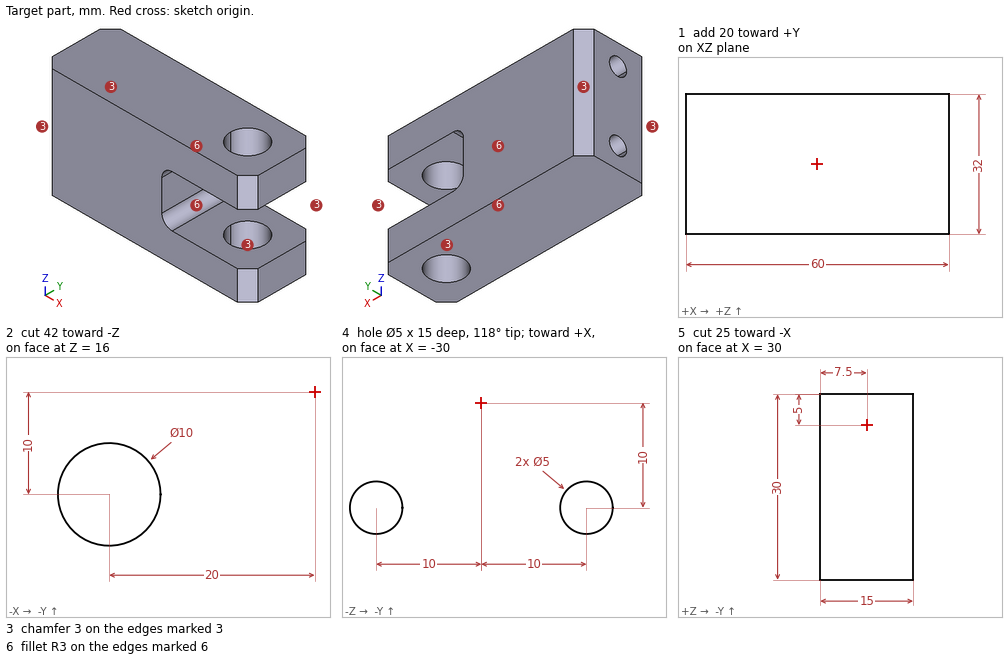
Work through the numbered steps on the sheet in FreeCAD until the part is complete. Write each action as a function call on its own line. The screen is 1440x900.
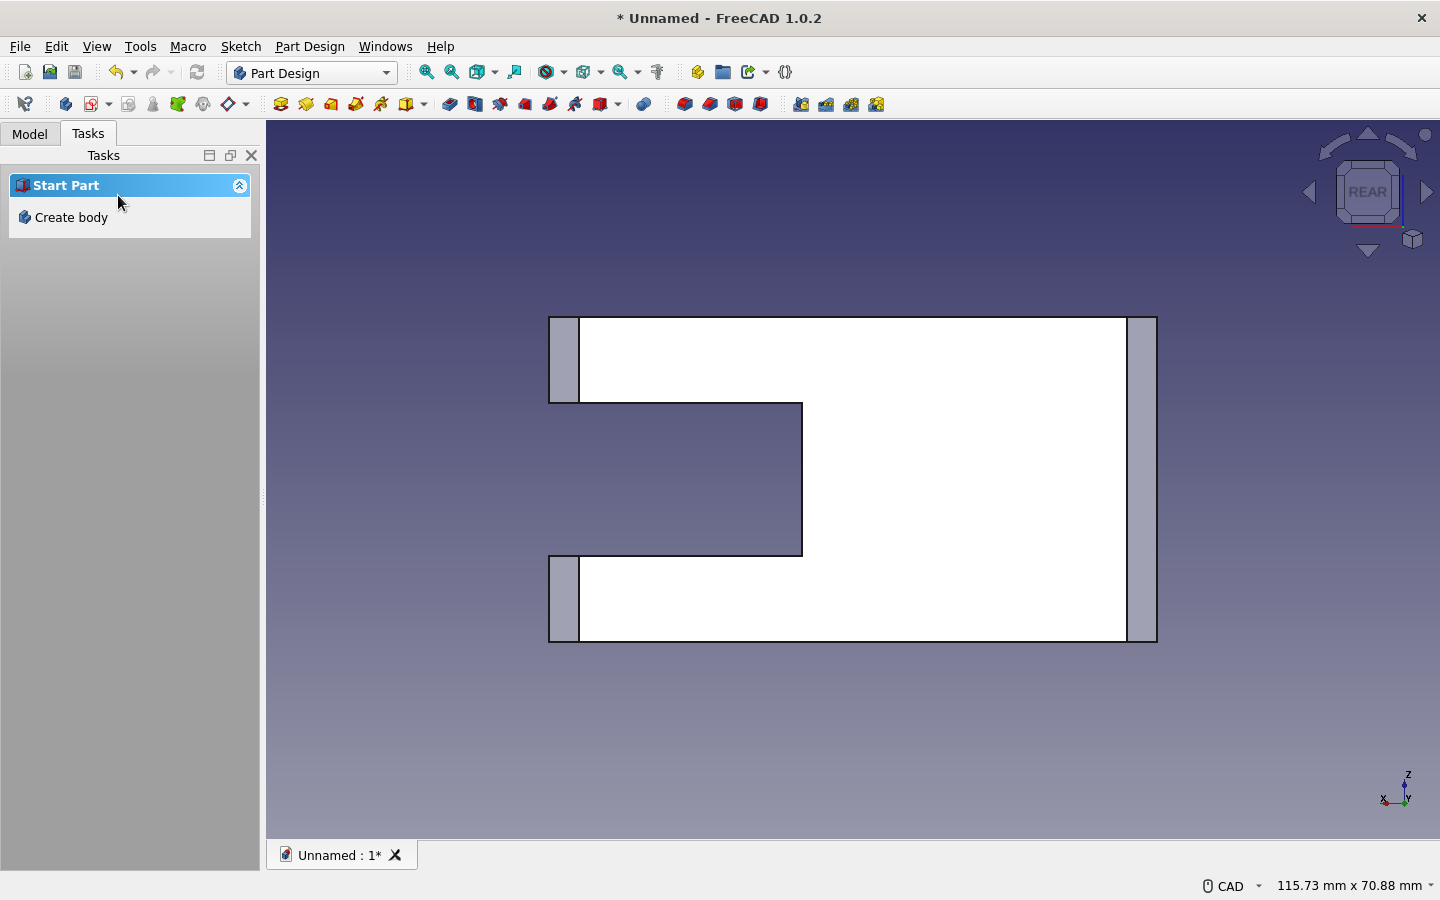
key(6)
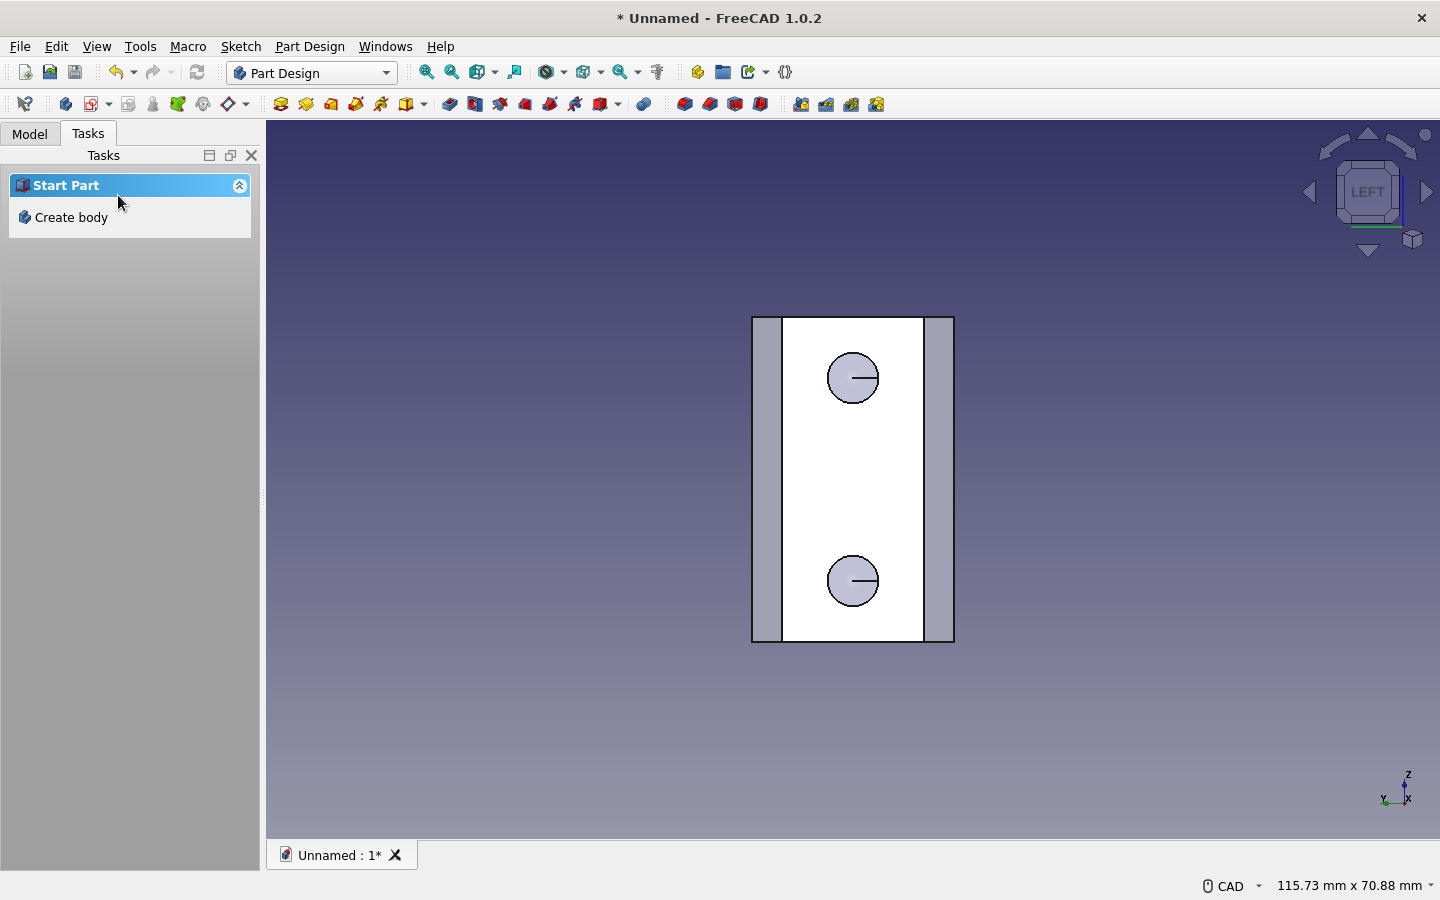
key(v)
key(3)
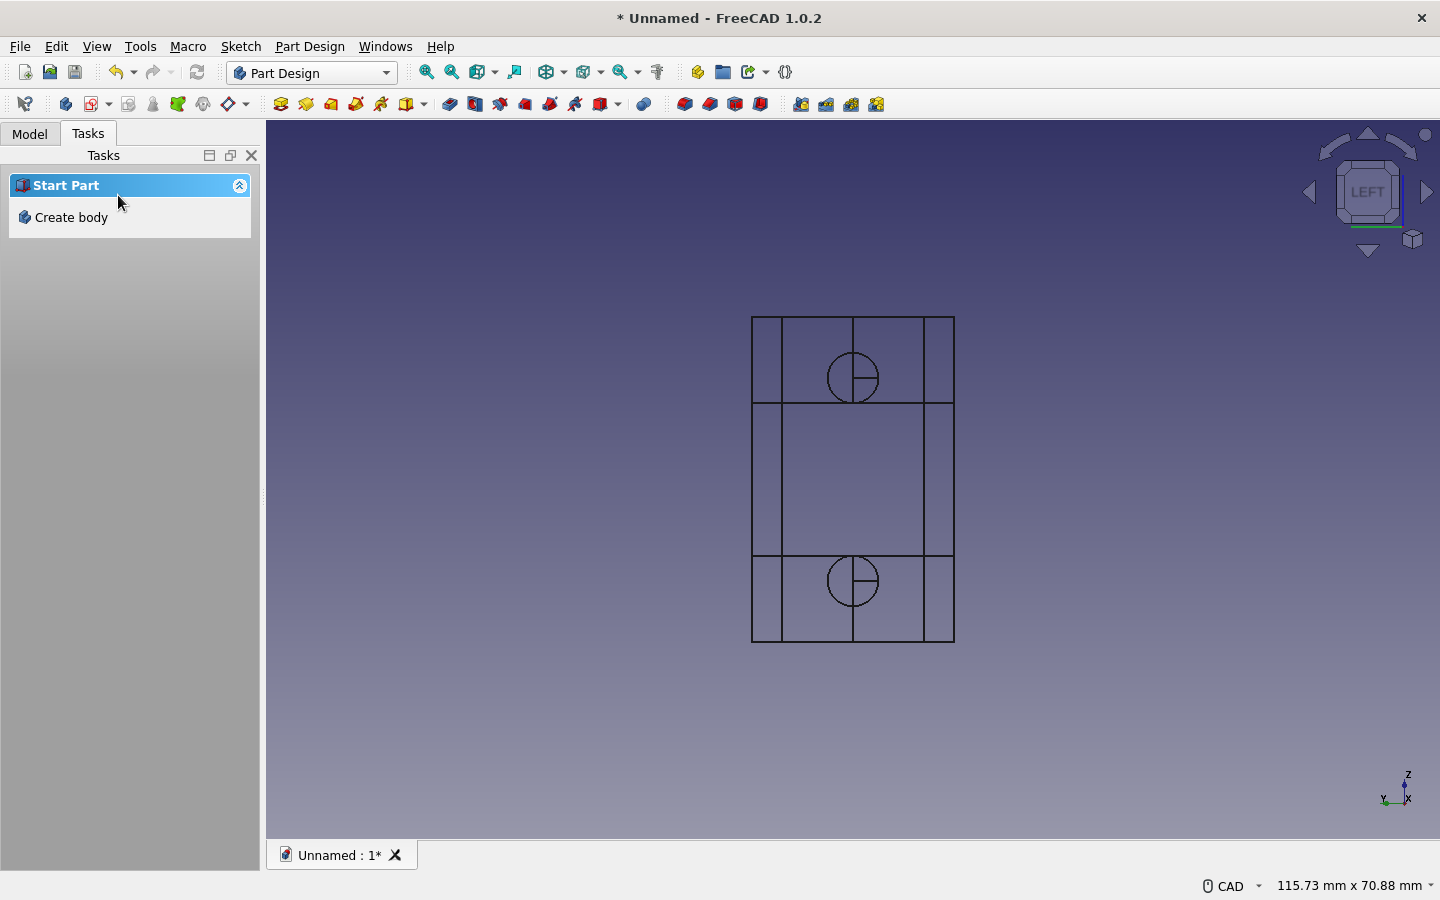
key(0)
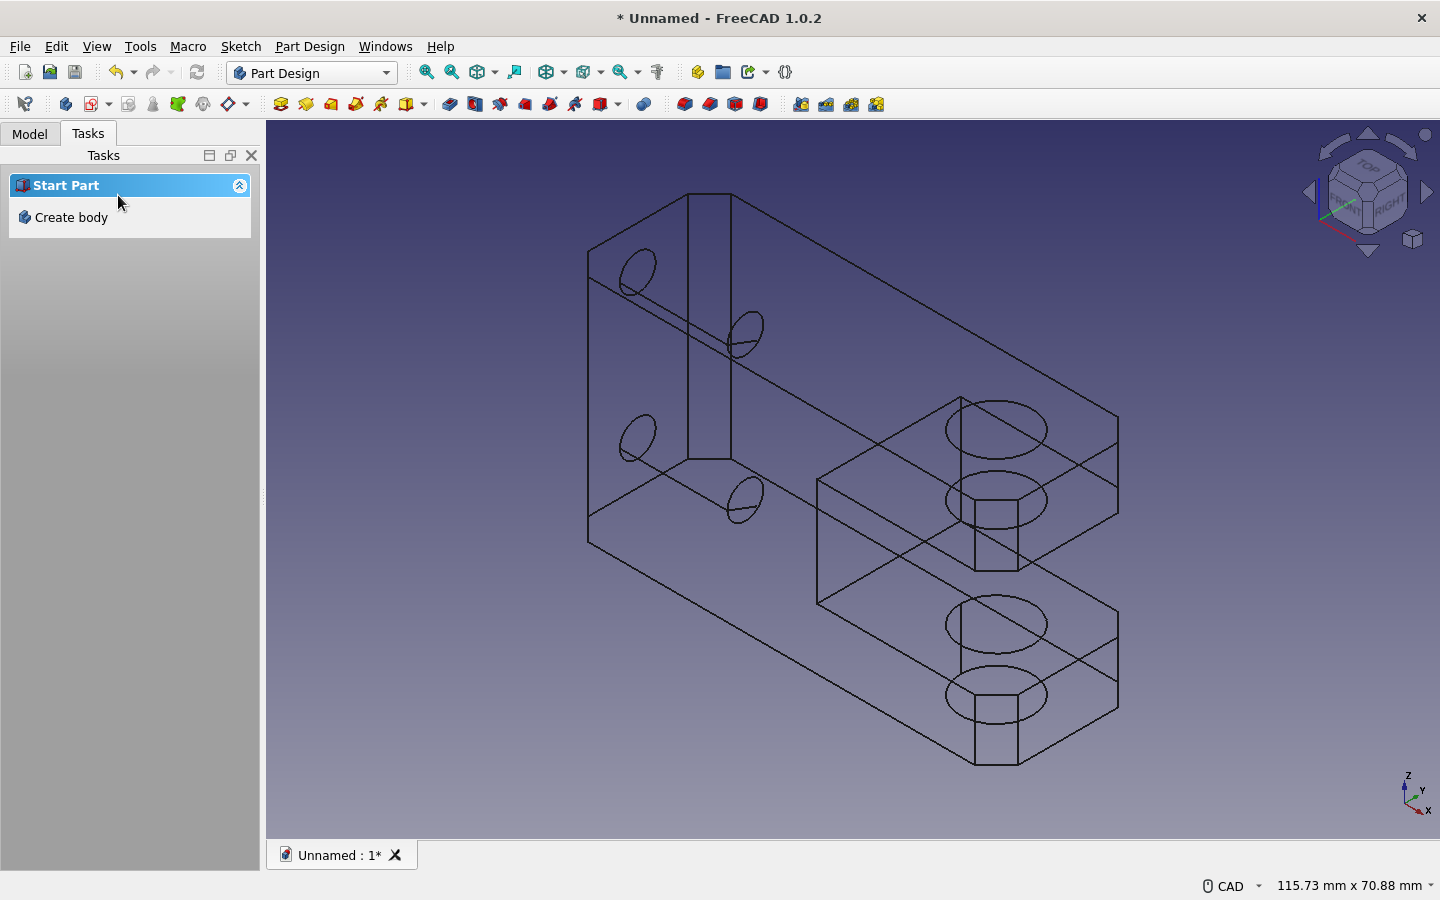
click(889, 561)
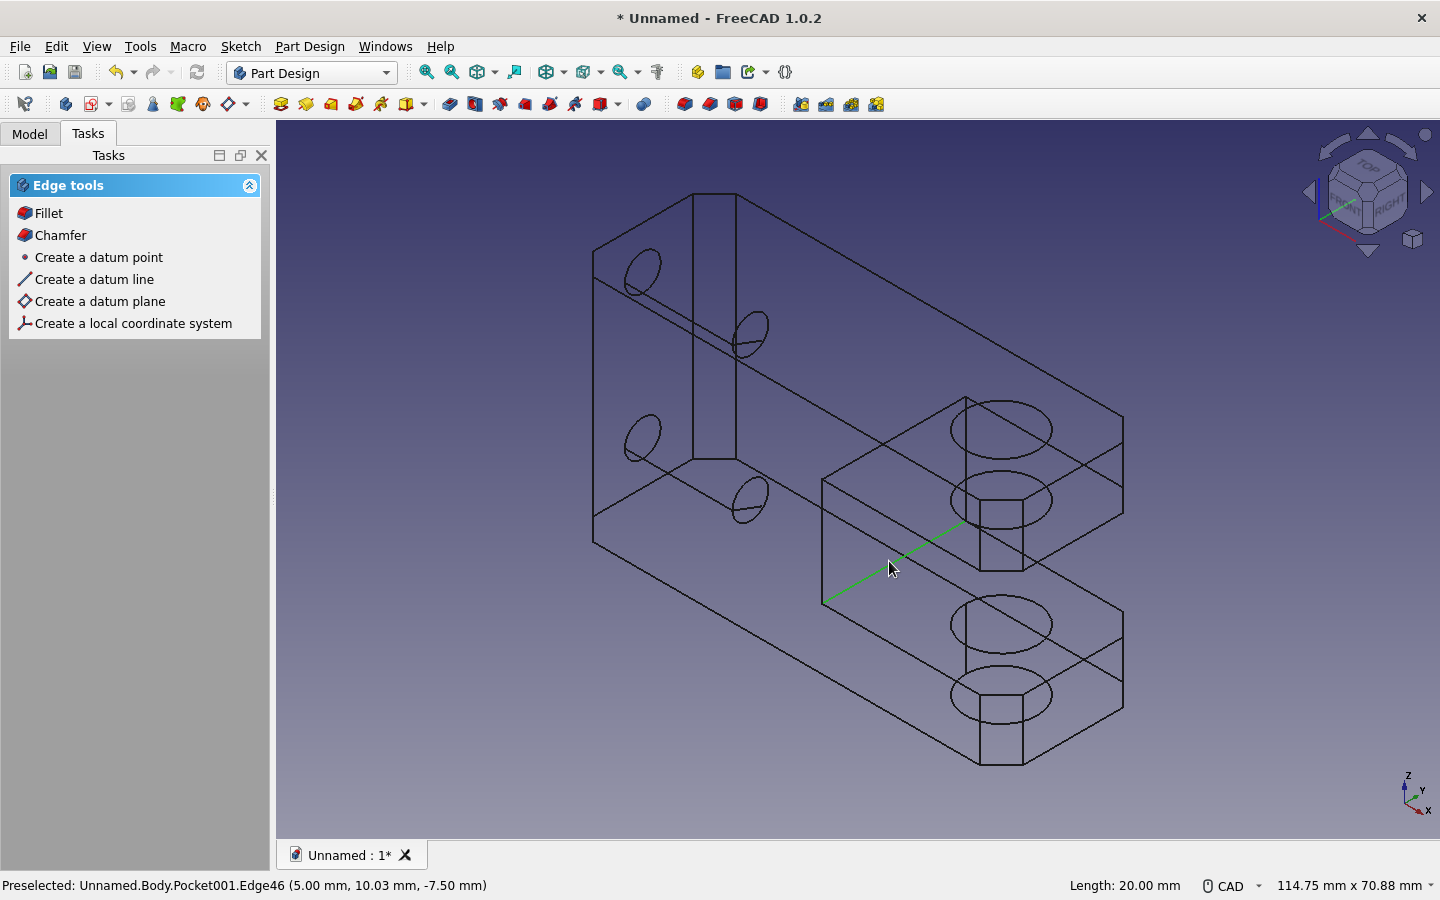
click(894, 437, ctrl)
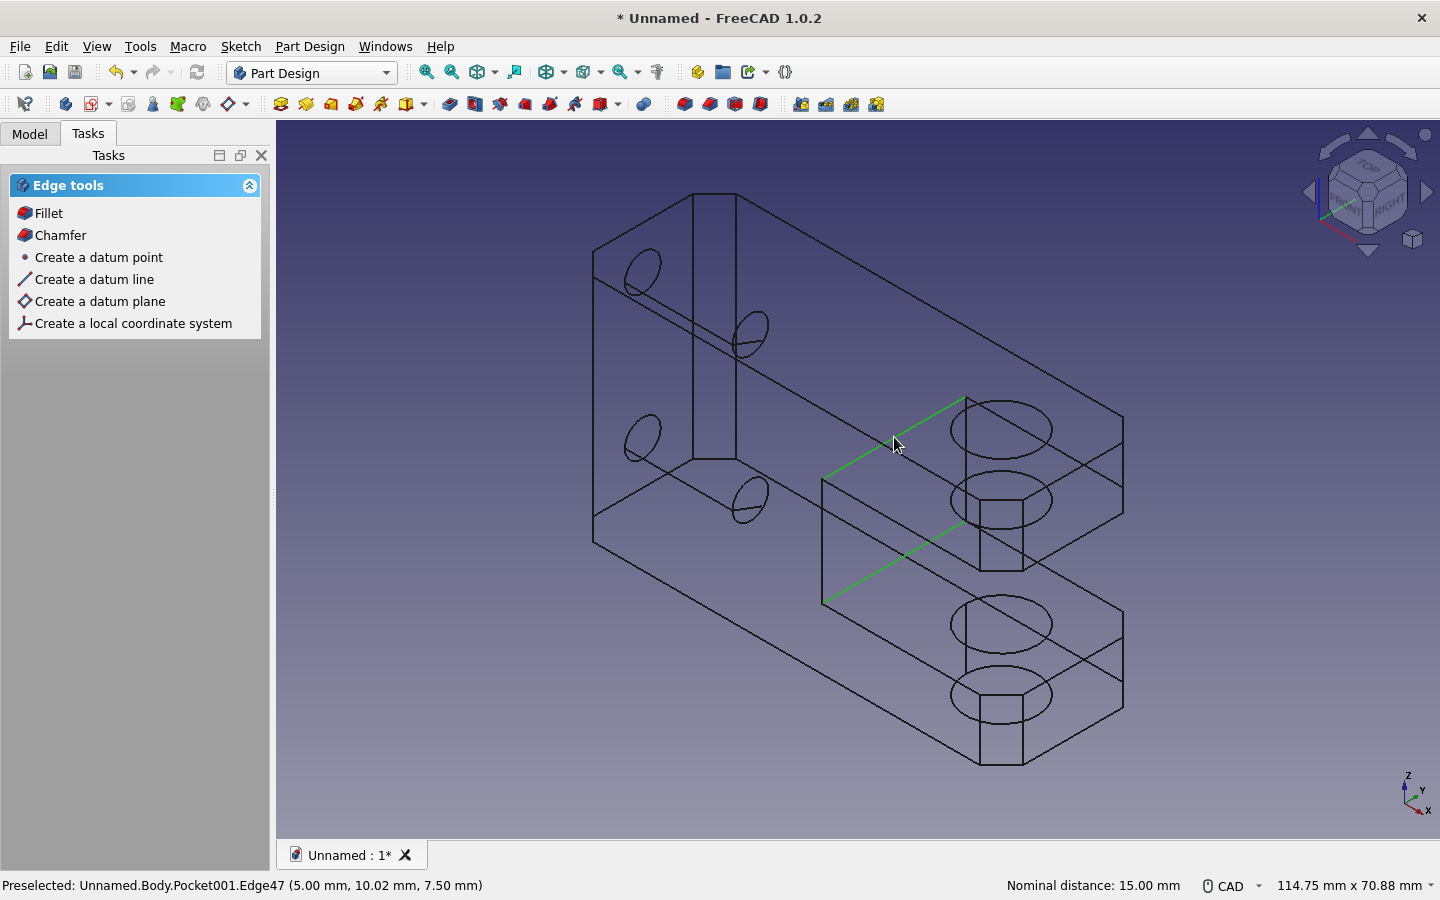
key(v)
key(1)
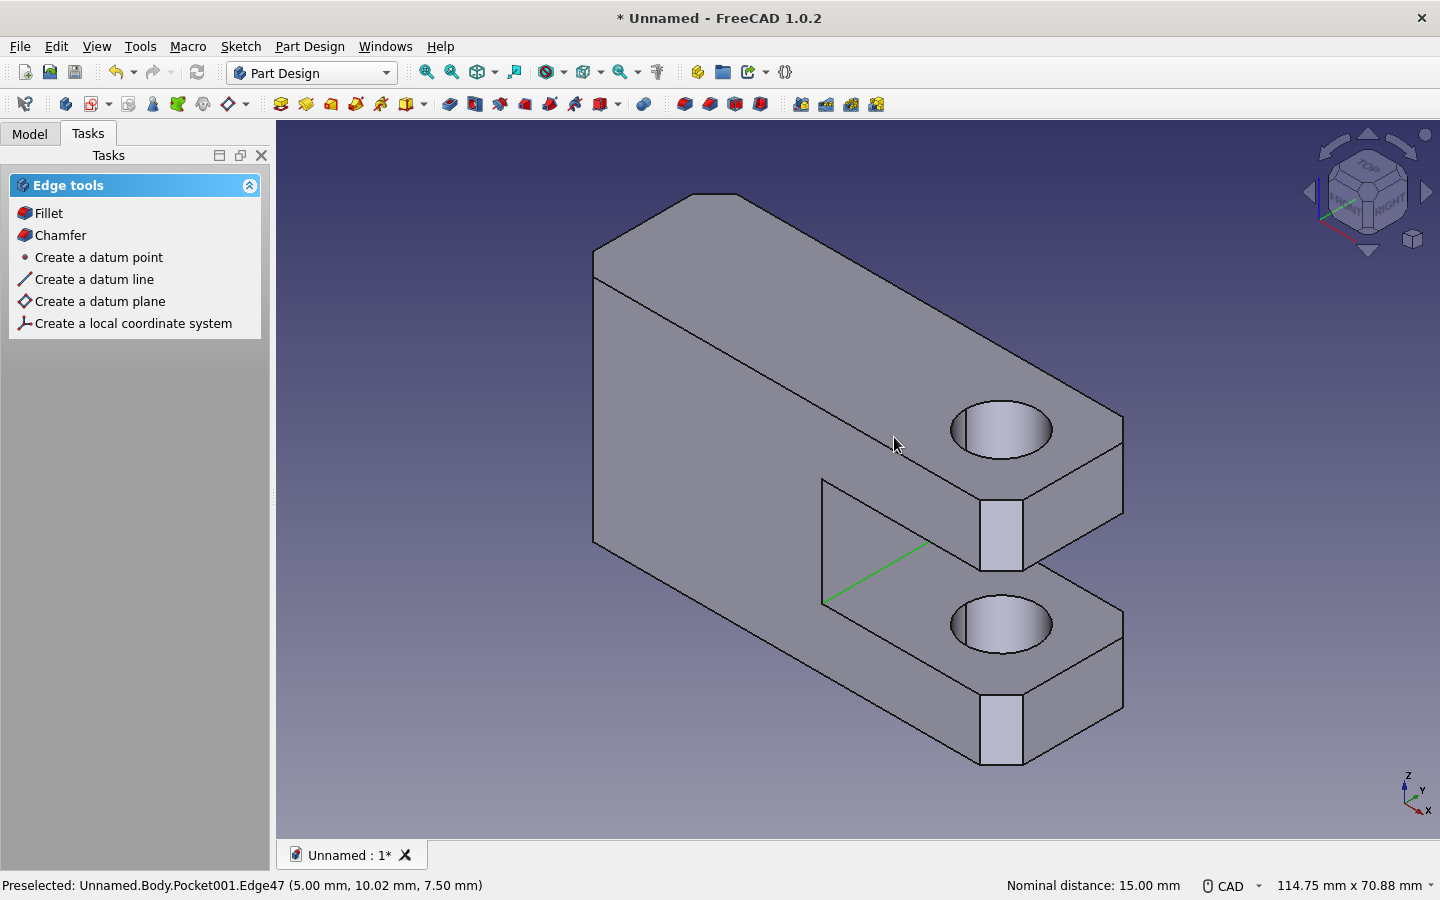
click(685, 104)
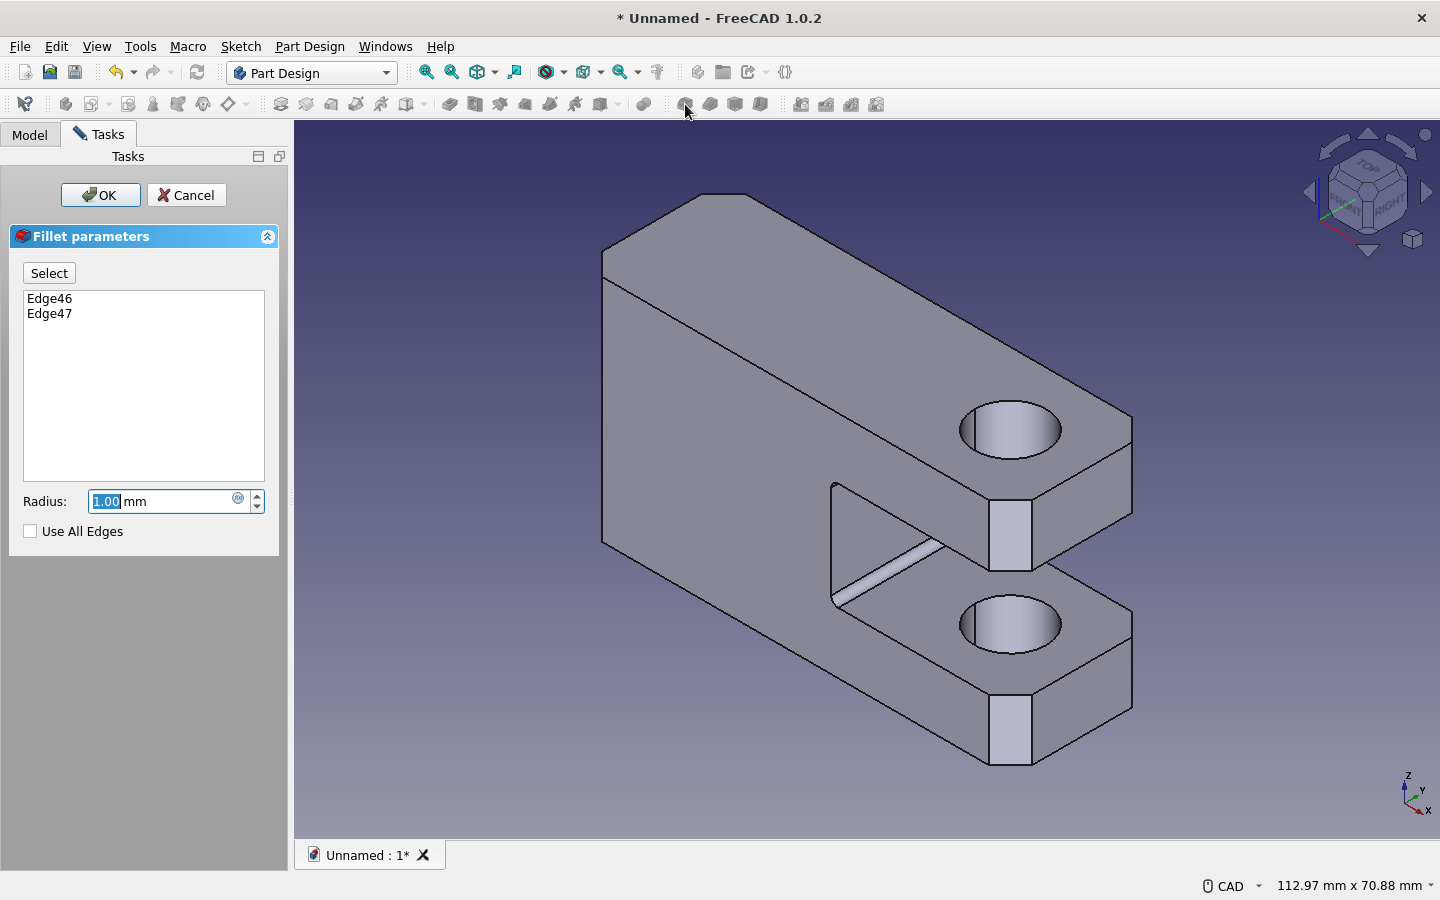
text(3)
key(Tab)